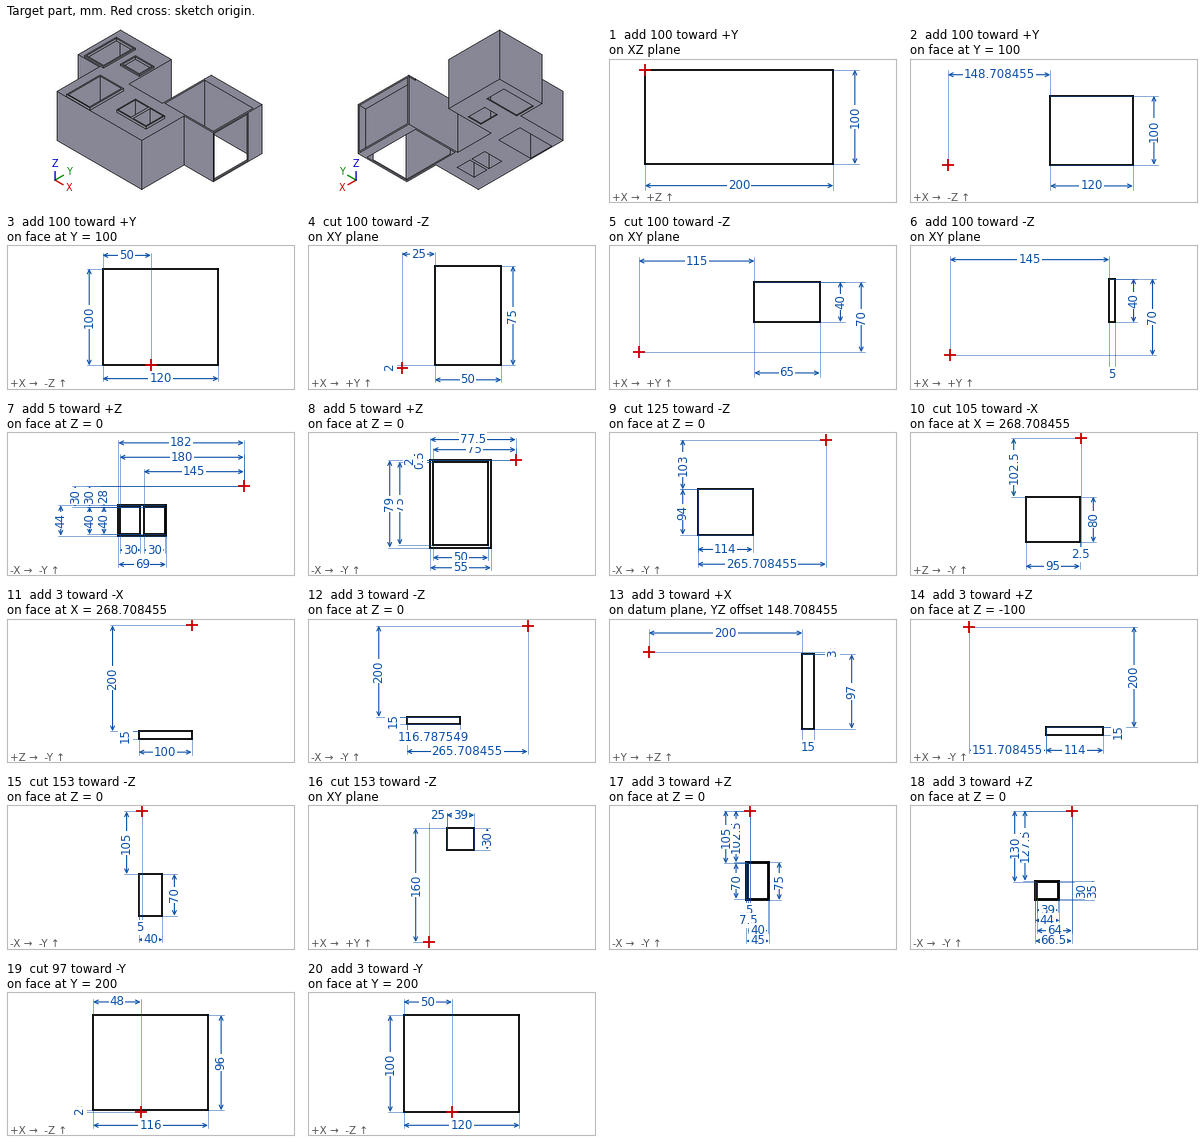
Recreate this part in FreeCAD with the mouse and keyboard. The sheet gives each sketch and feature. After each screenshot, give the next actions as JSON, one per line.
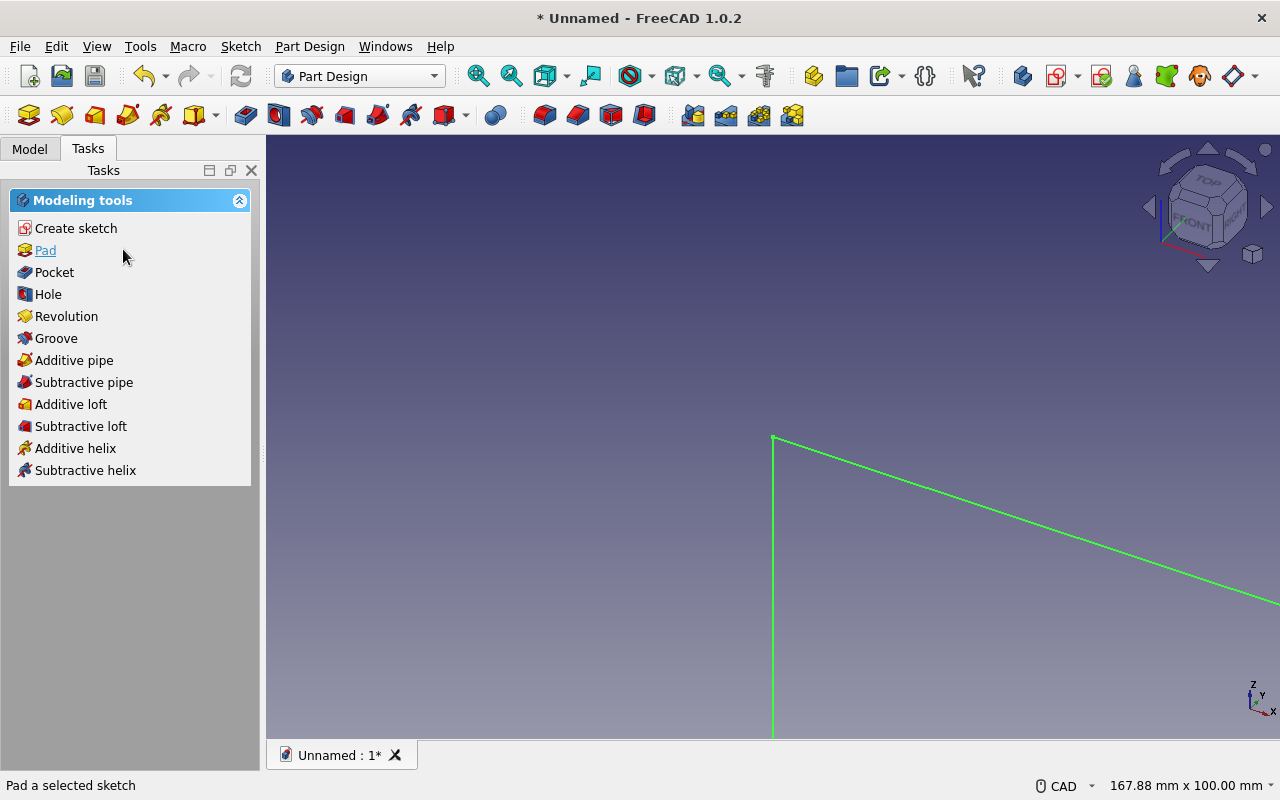
{"action": "left_click", "coordinate": [29, 116]}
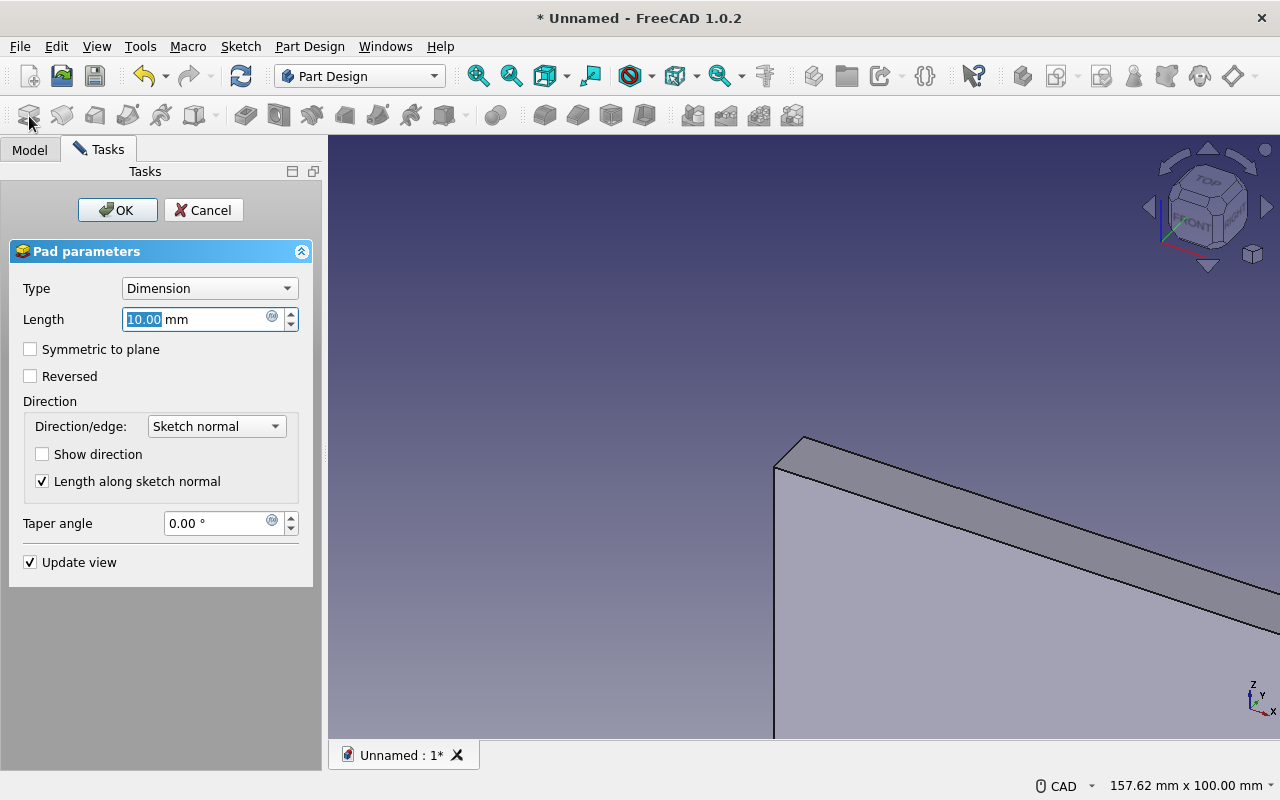
{"action": "type", "text": "100"}
{"action": "key", "text": "Tab"}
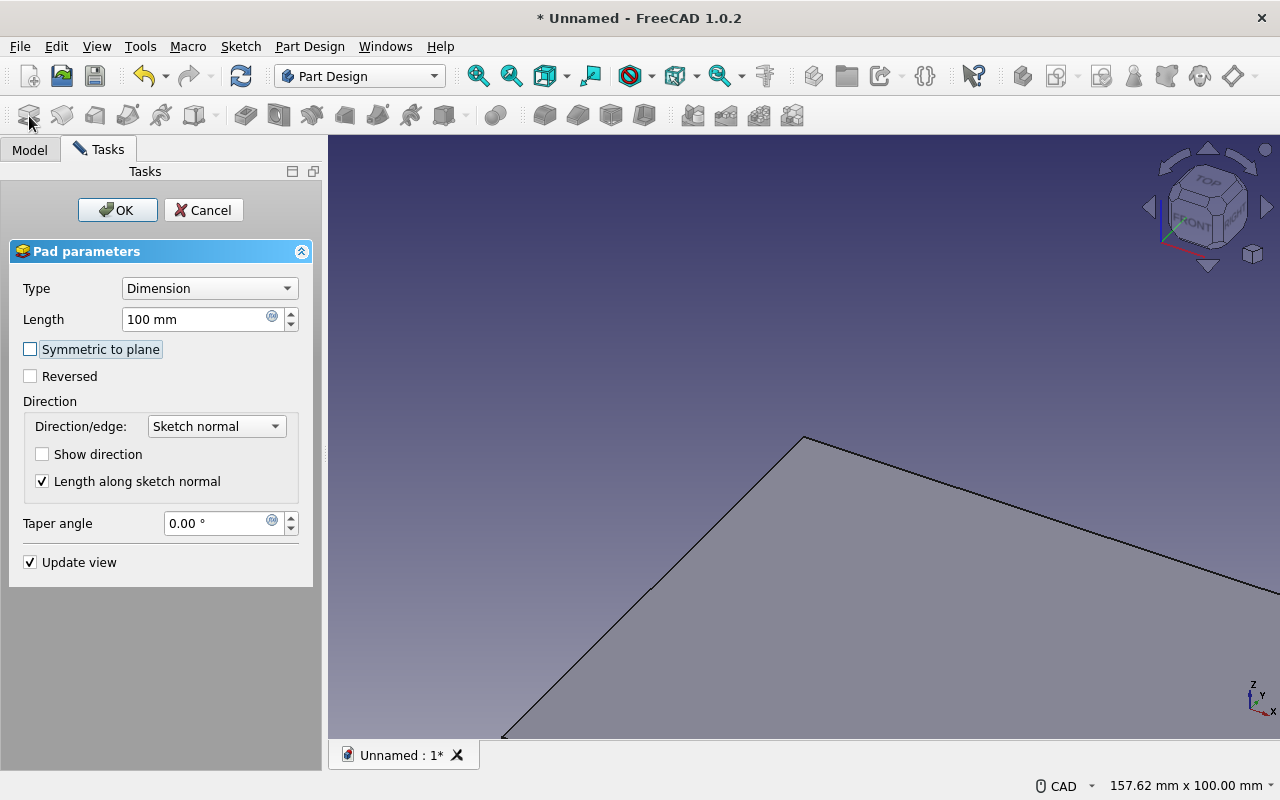
{"action": "left_click", "coordinate": [31, 376]}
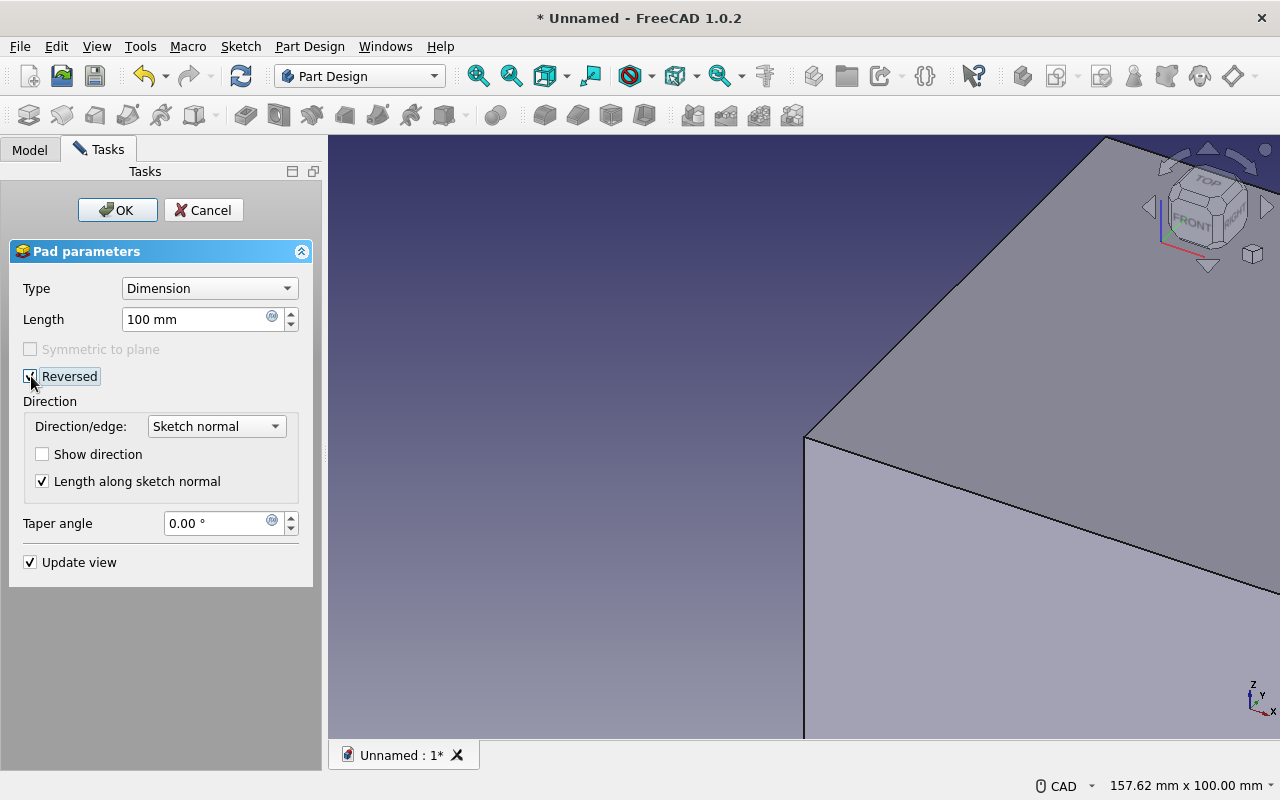
{"action": "left_click", "coordinate": [118, 210]}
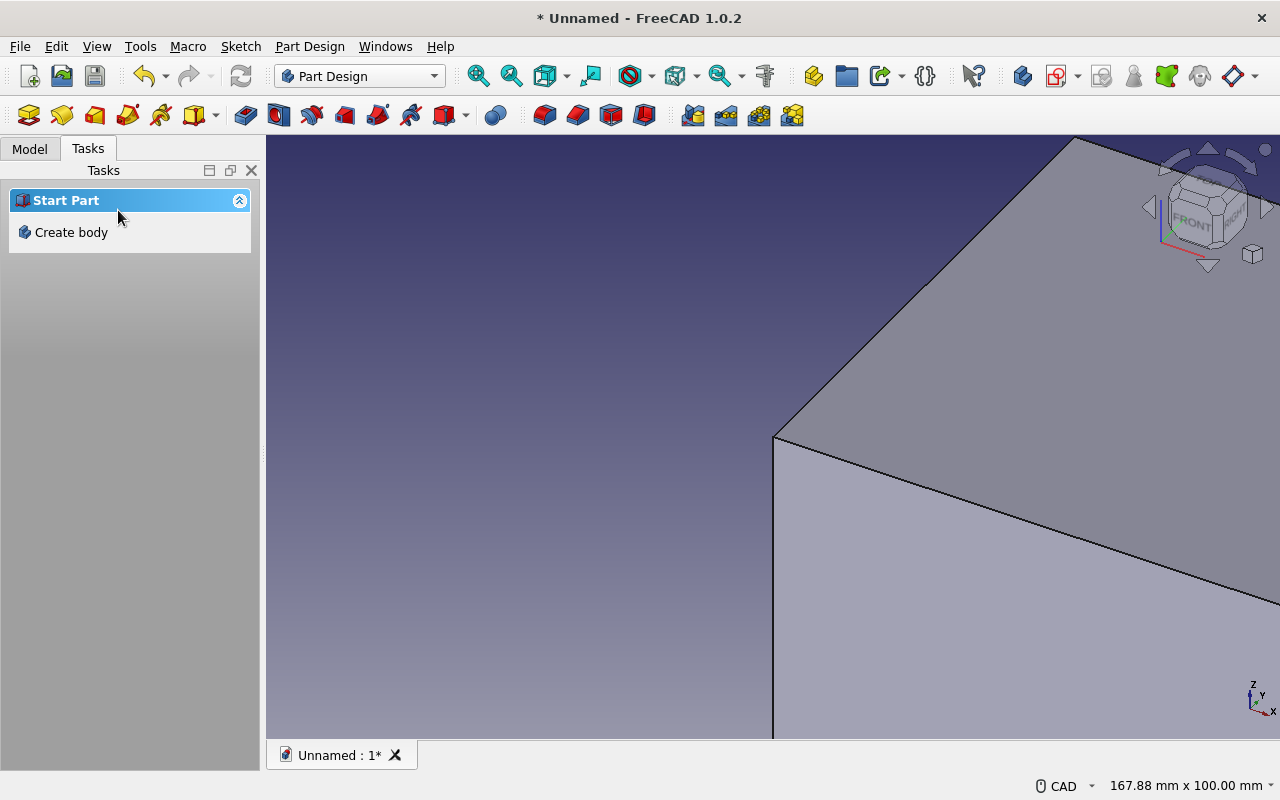
{"action": "left_click", "coordinate": [479, 76]}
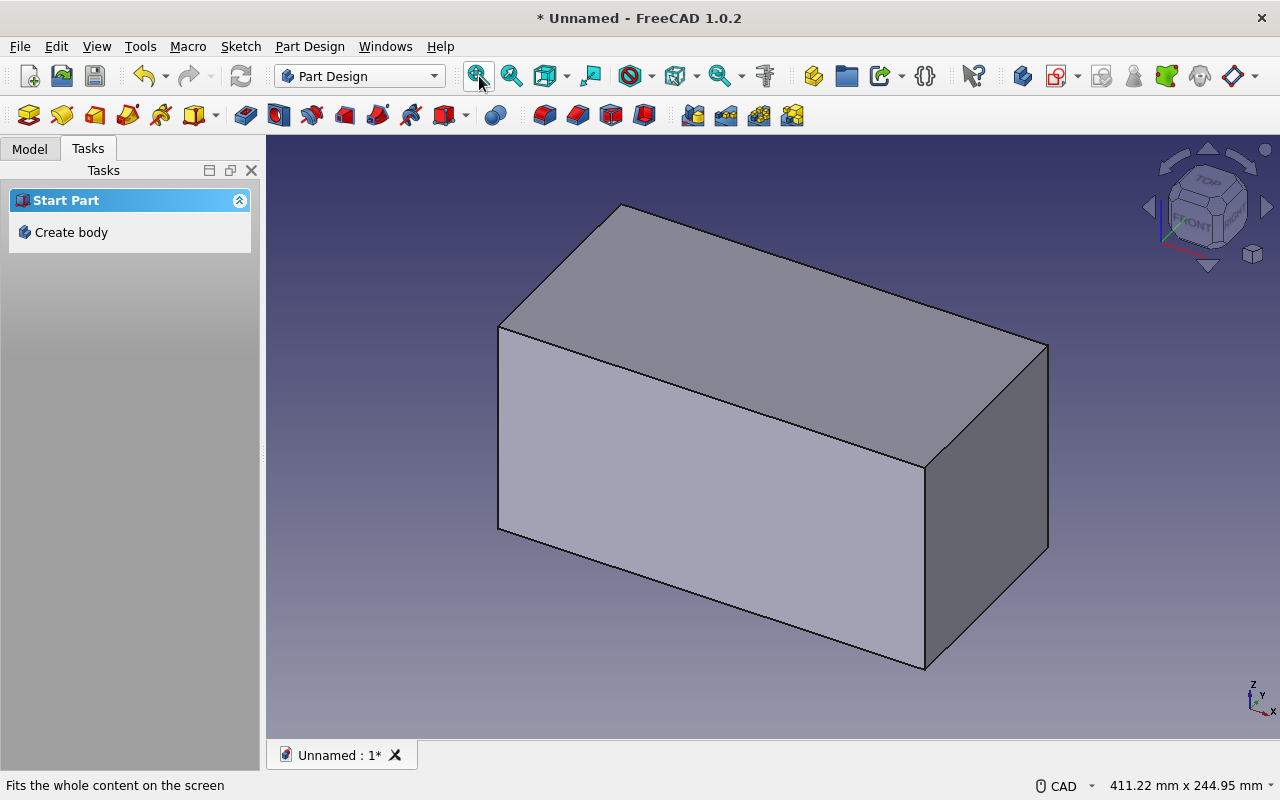
{"action": "key", "text": "4"}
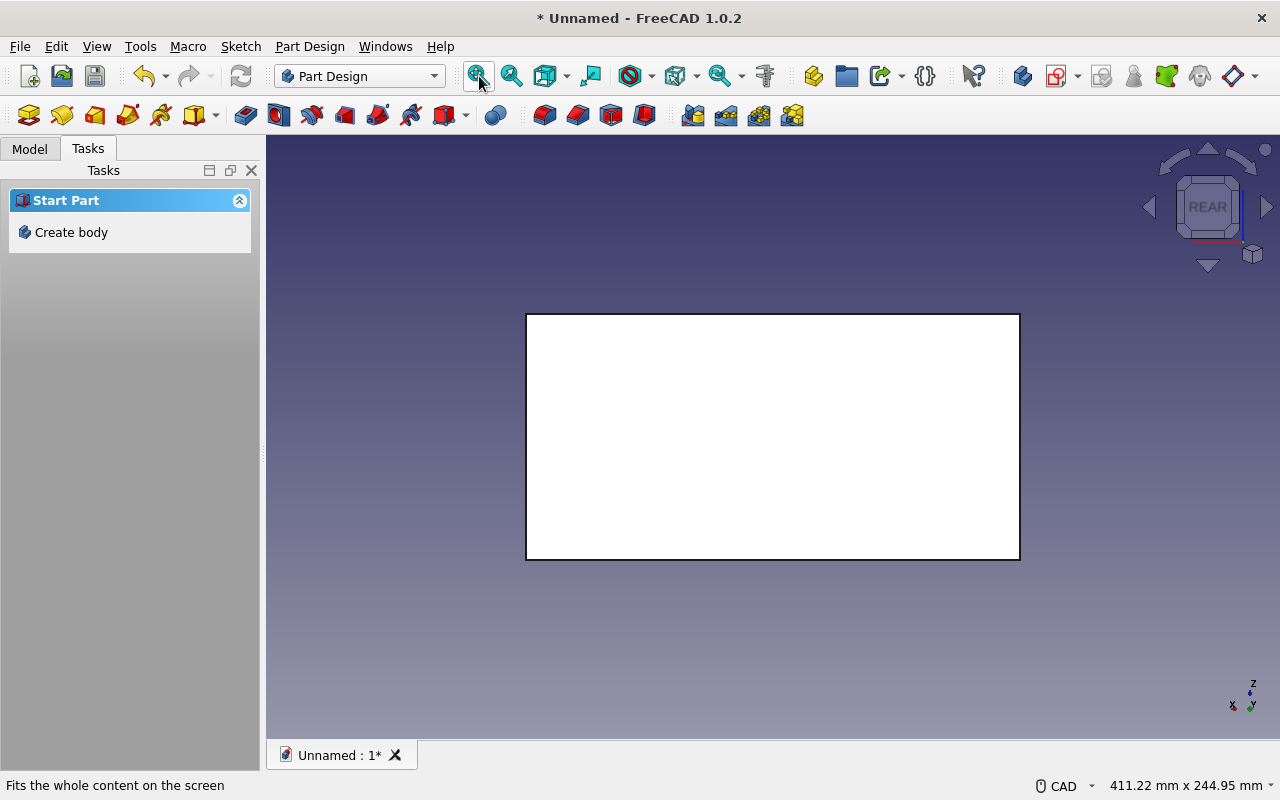
{"action": "left_click", "coordinate": [703, 436]}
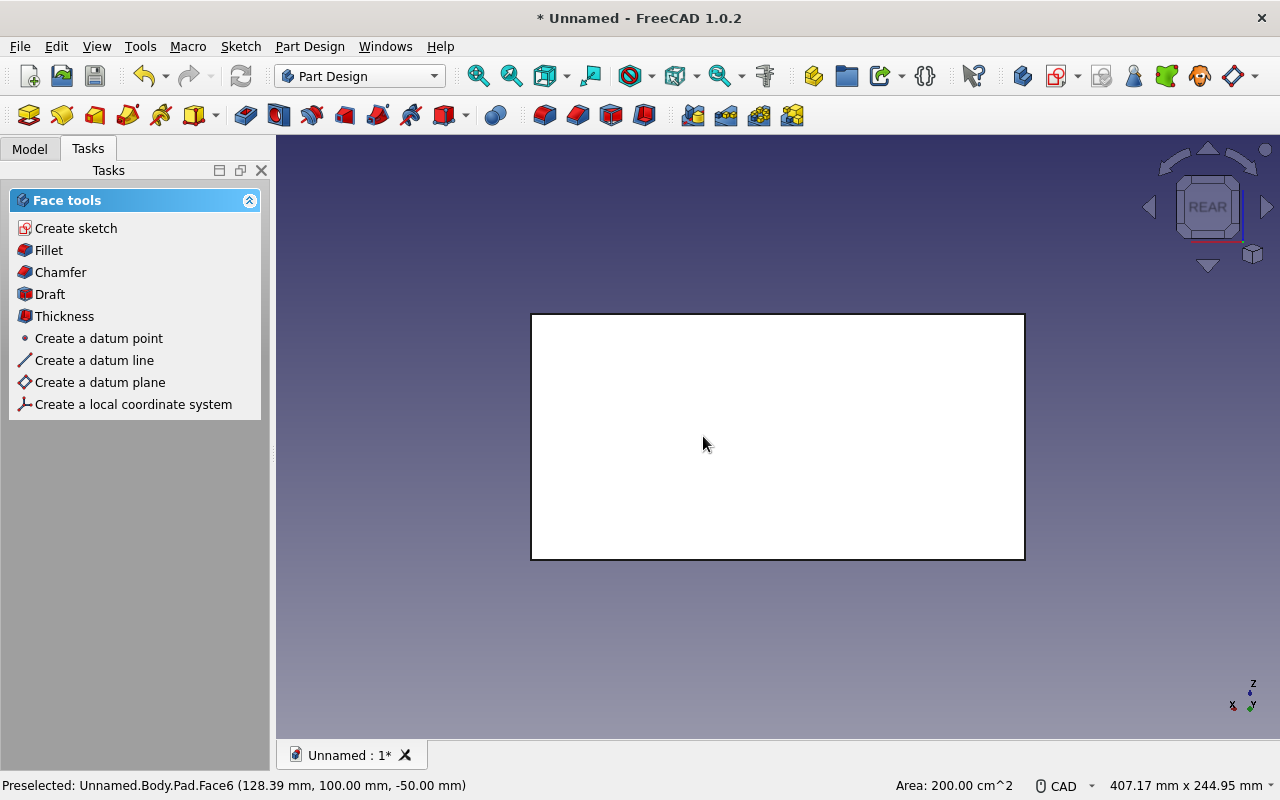
{"action": "left_click", "coordinate": [1056, 76]}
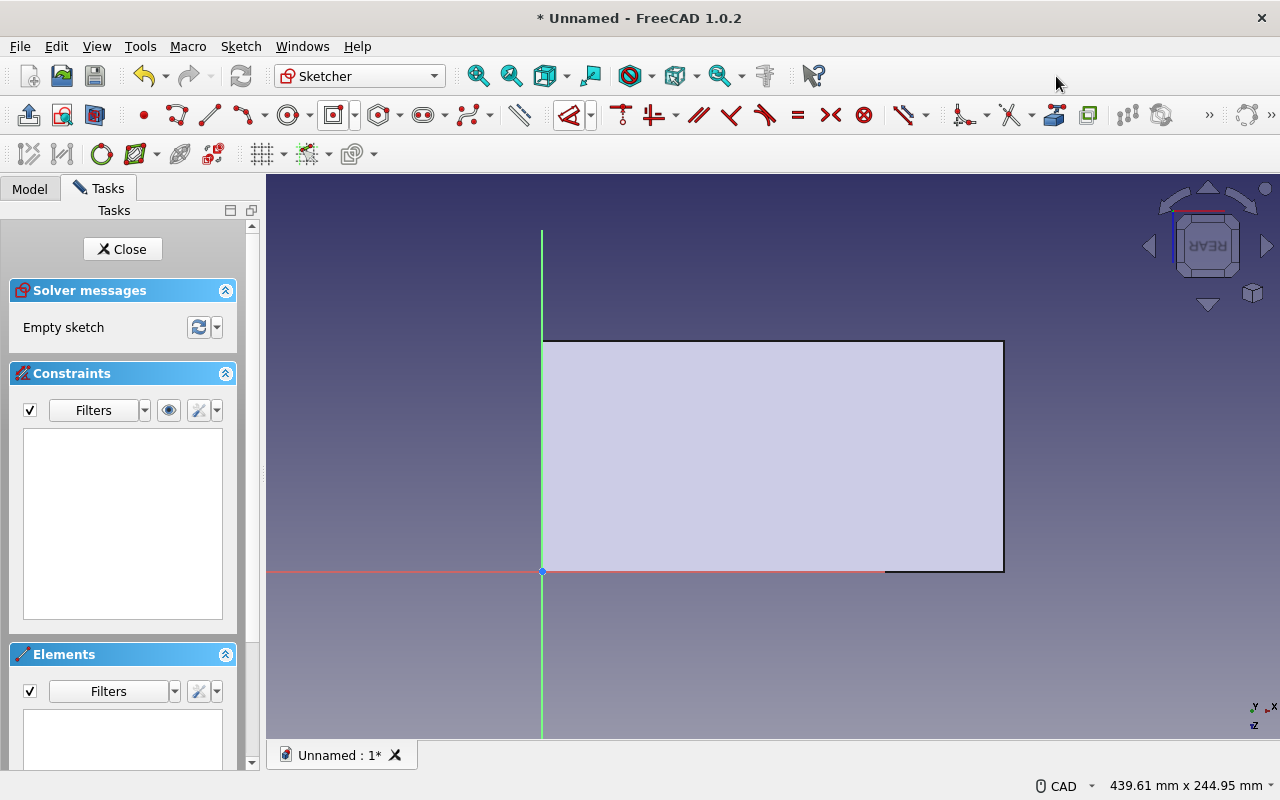
{"action": "scroll", "coordinate": [294, 457], "scroll_direction": "down", "scroll_amount": 1}